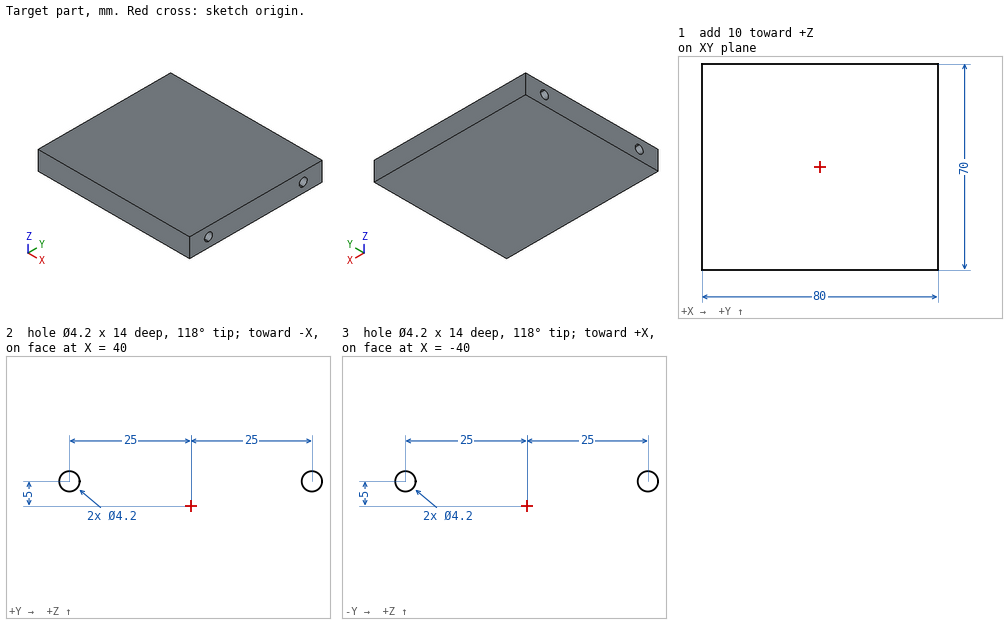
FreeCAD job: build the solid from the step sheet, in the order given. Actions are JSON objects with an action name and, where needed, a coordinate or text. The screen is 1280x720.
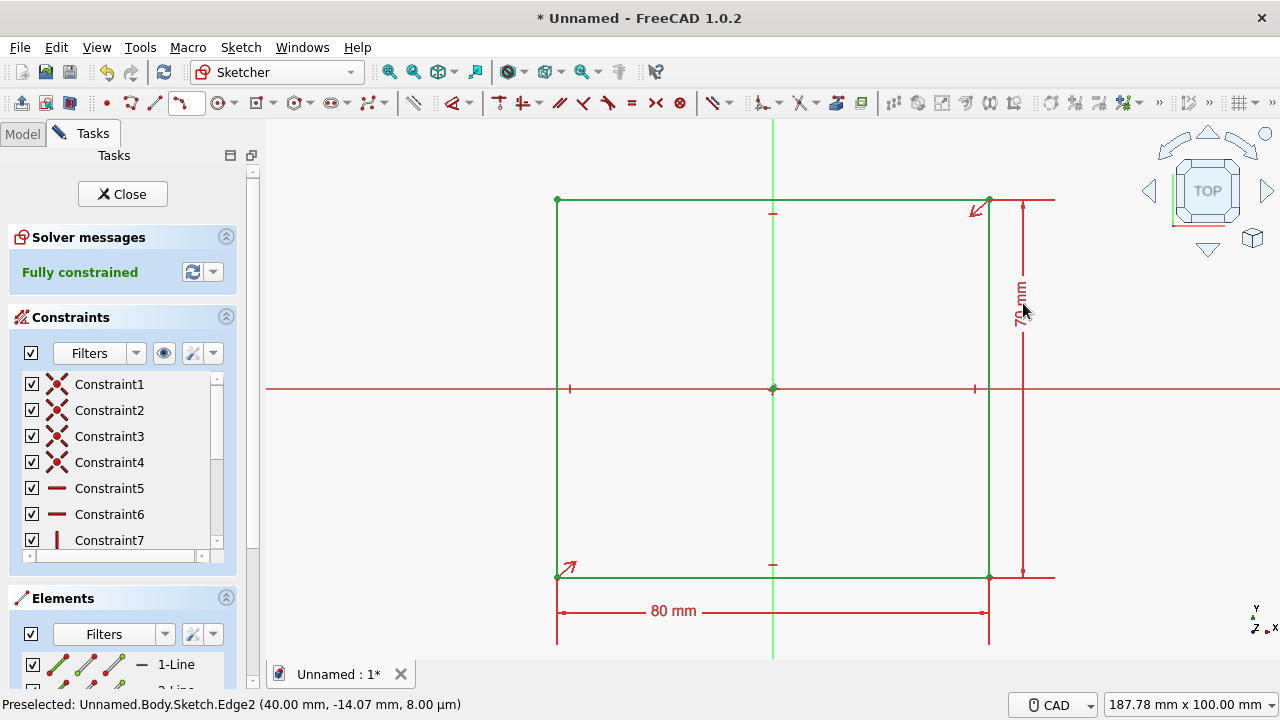
{"action": "left_click", "coordinate": [123, 194]}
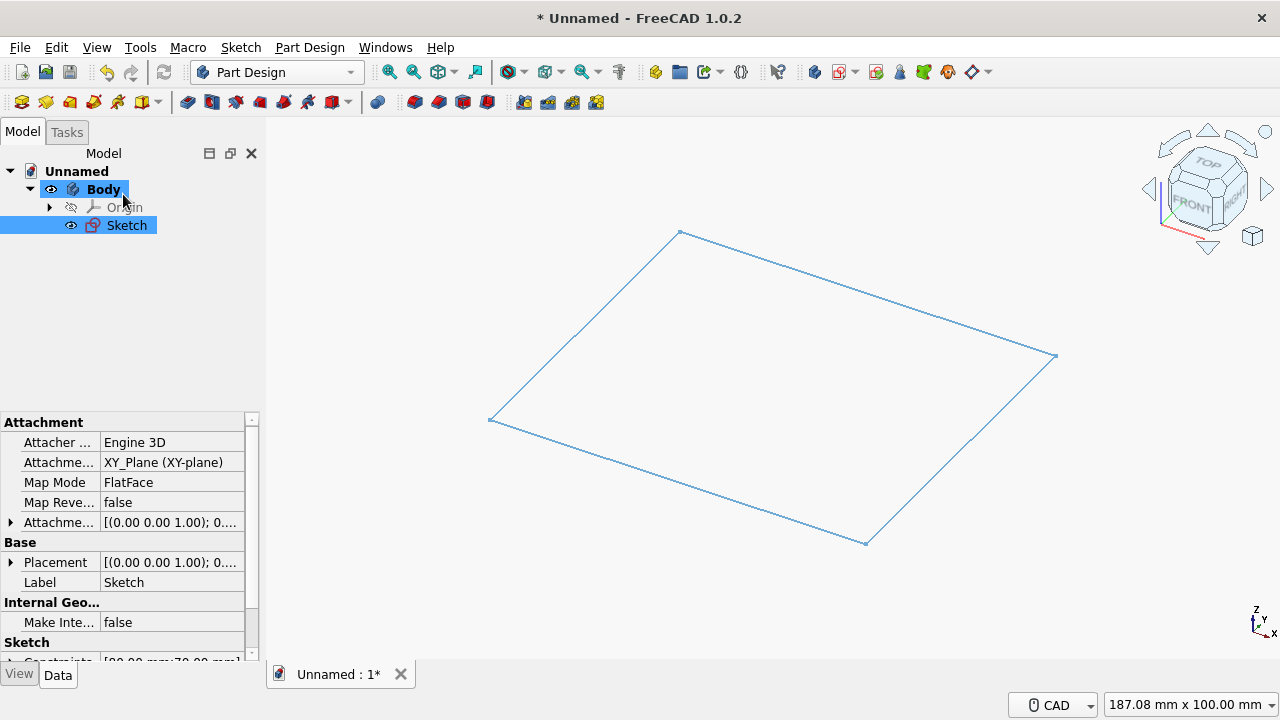
{"action": "left_click", "coordinate": [22, 102]}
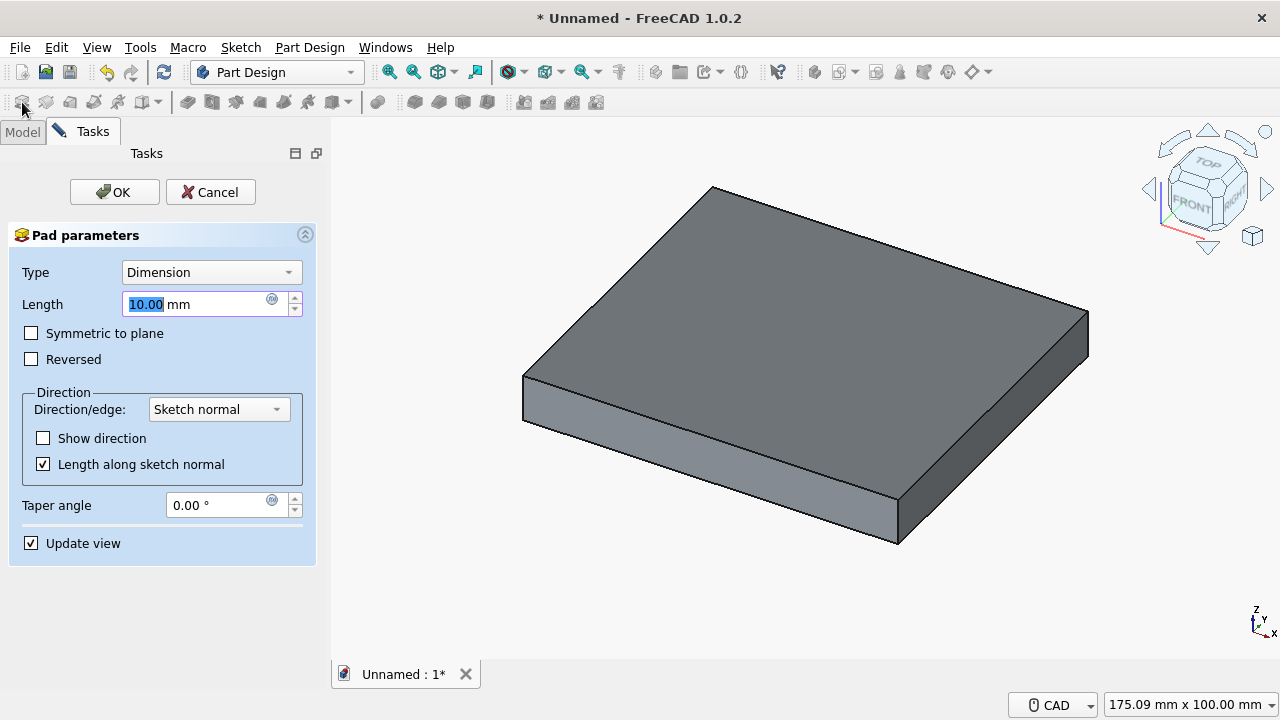
{"action": "type", "text": "10"}
{"action": "key", "text": "Tab"}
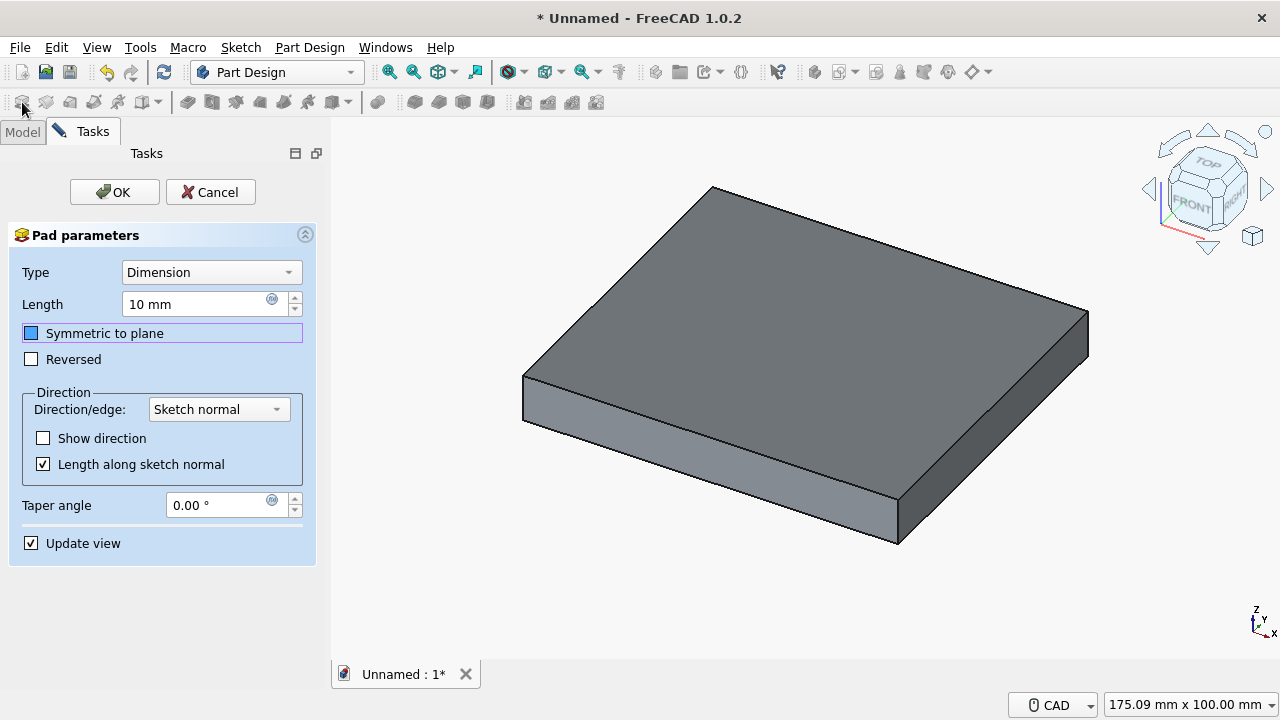
{"action": "left_click", "coordinate": [115, 192]}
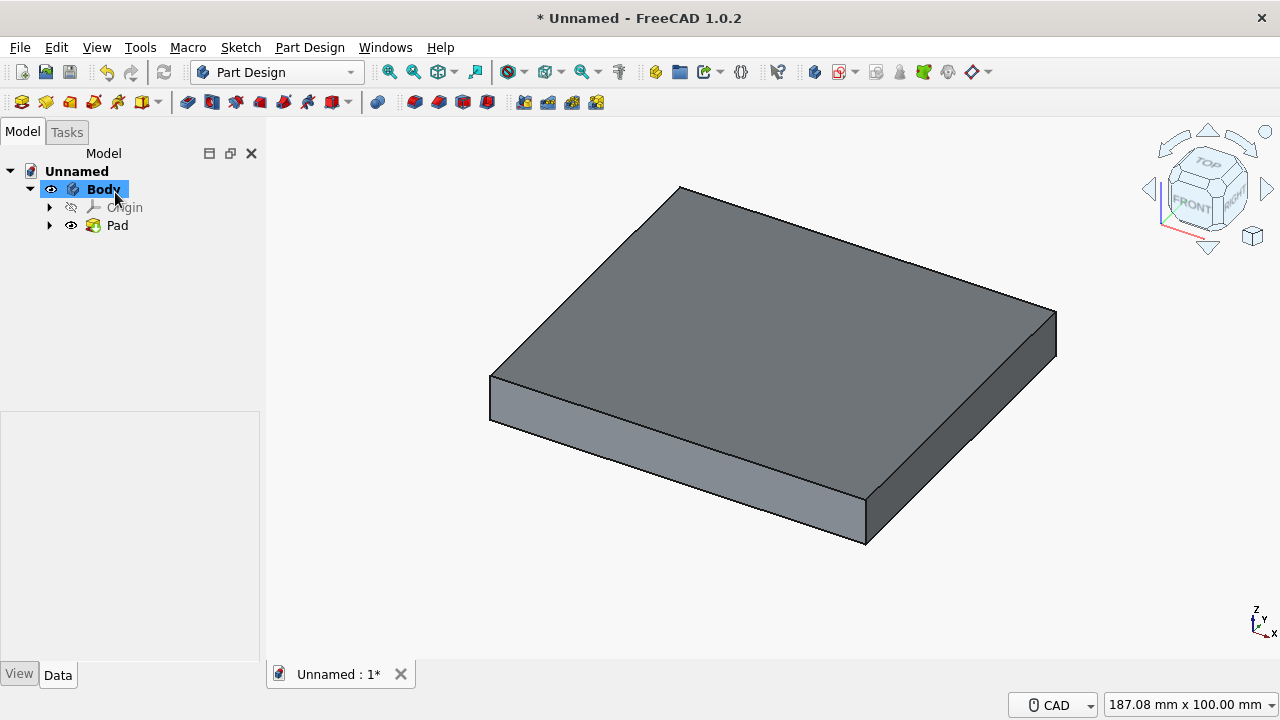
{"action": "left_click", "coordinate": [1042, 346]}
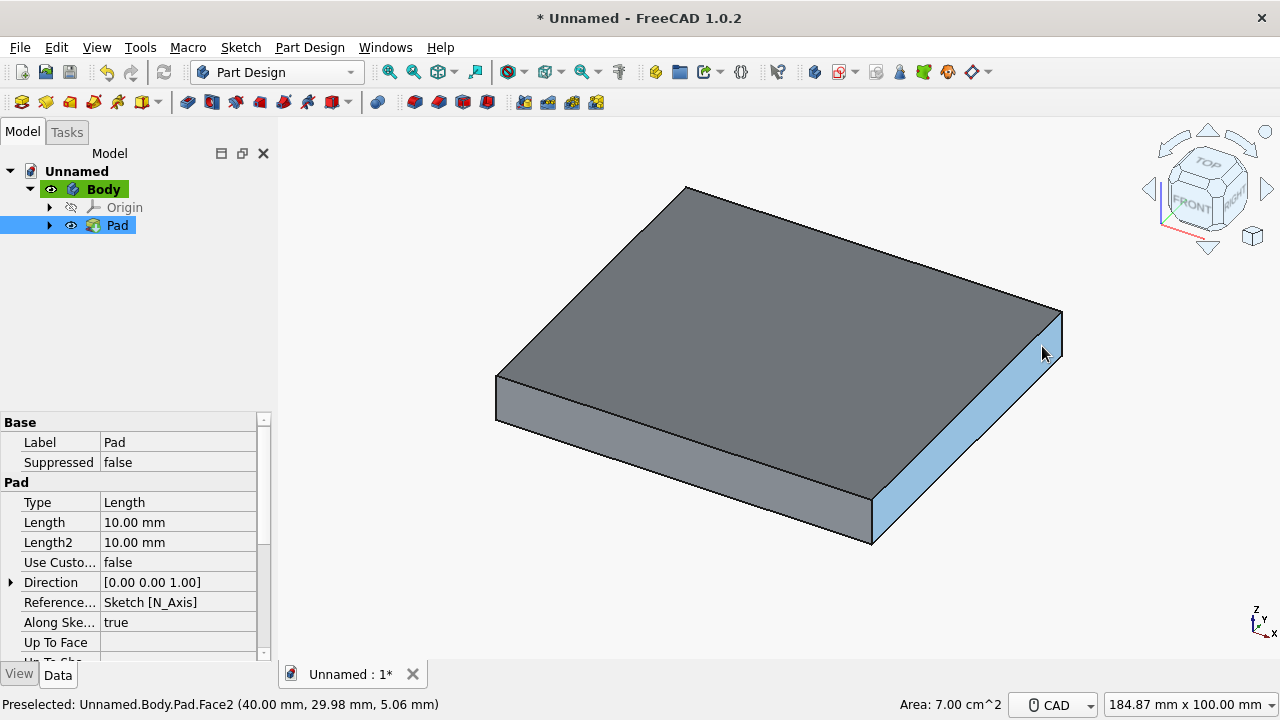
{"action": "left_click", "coordinate": [840, 72]}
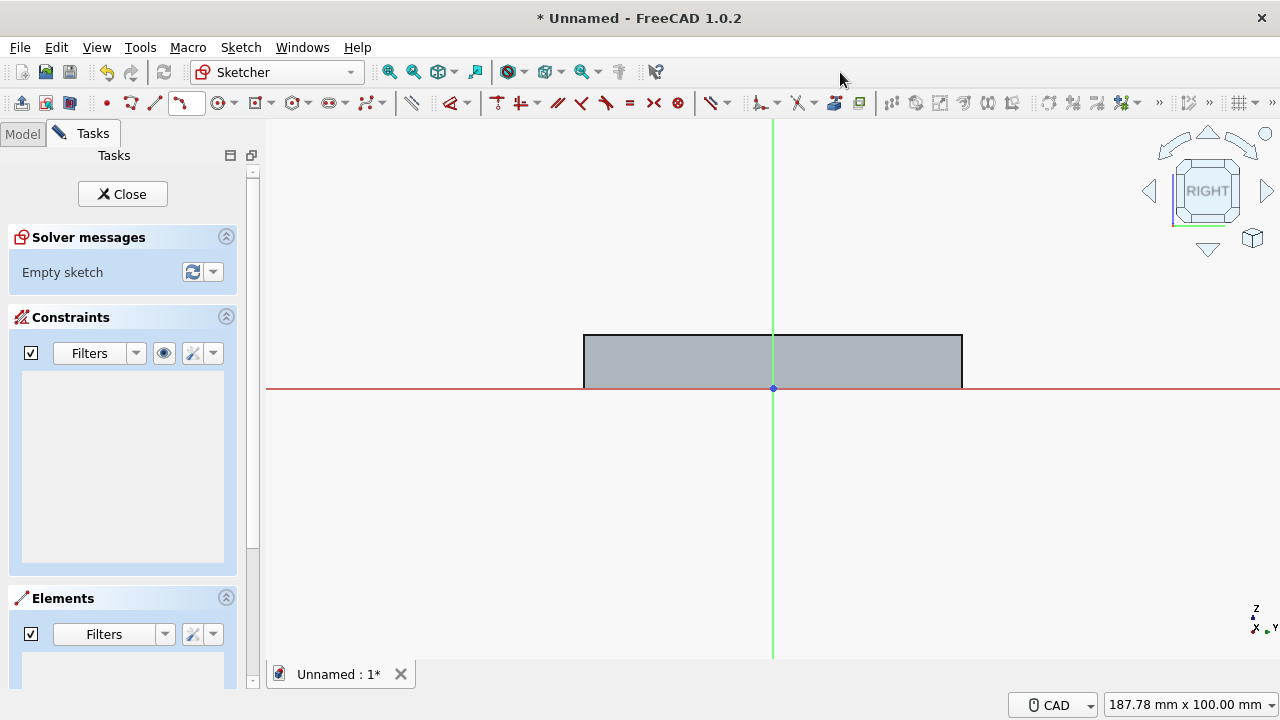
{"action": "scroll", "coordinate": [856, 347], "scroll_direction": "up", "scroll_amount": 3}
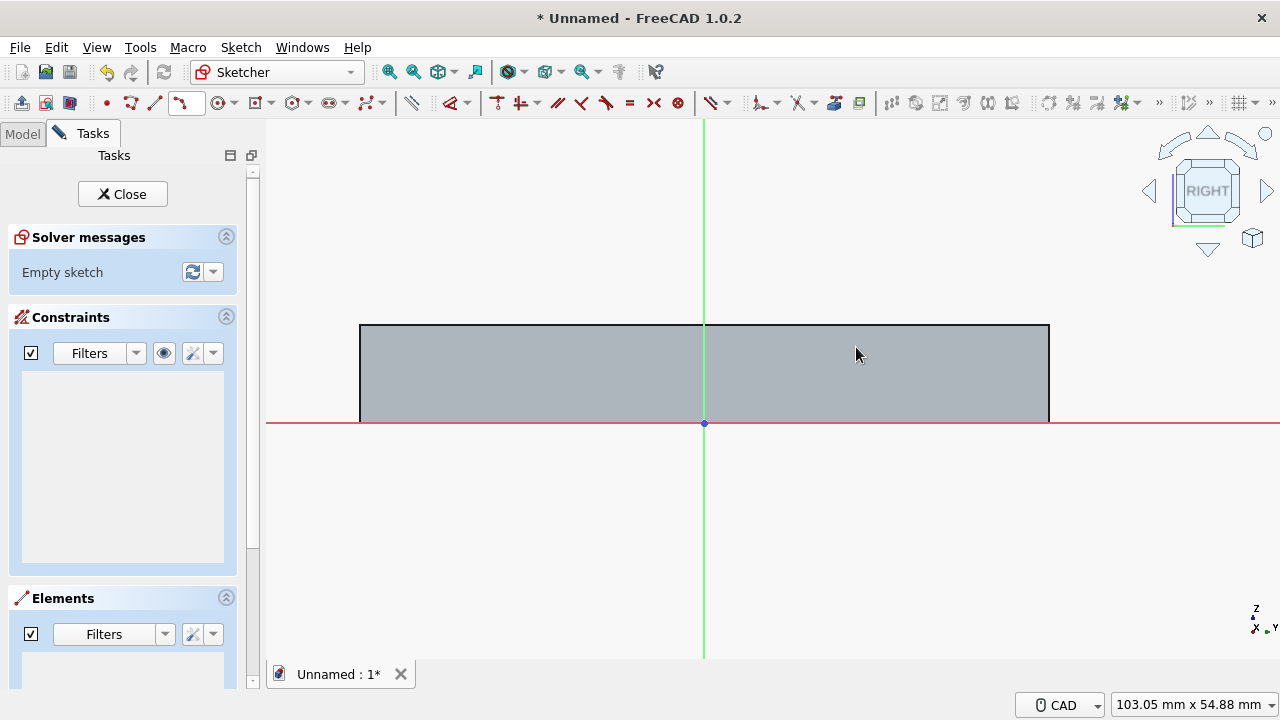
{"action": "left_click", "coordinate": [218, 104]}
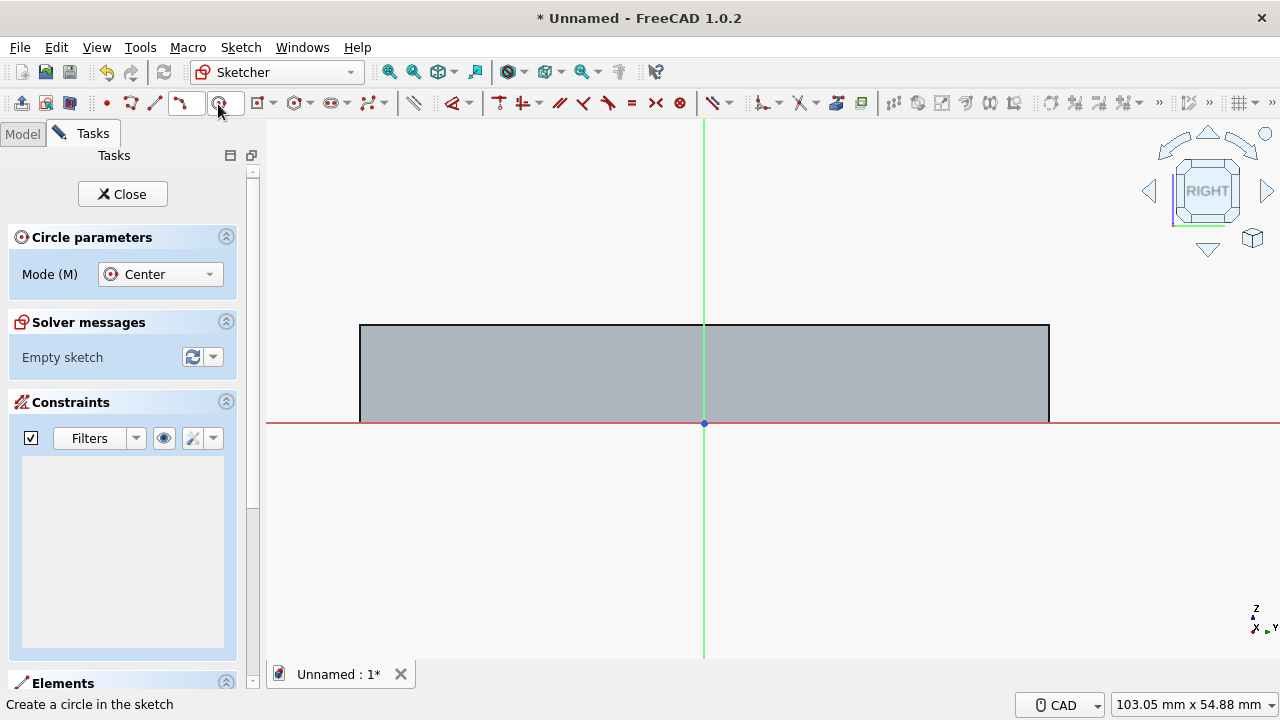
{"action": "left_click", "coordinate": [458, 374]}
{"action": "left_click", "coordinate": [473, 359]}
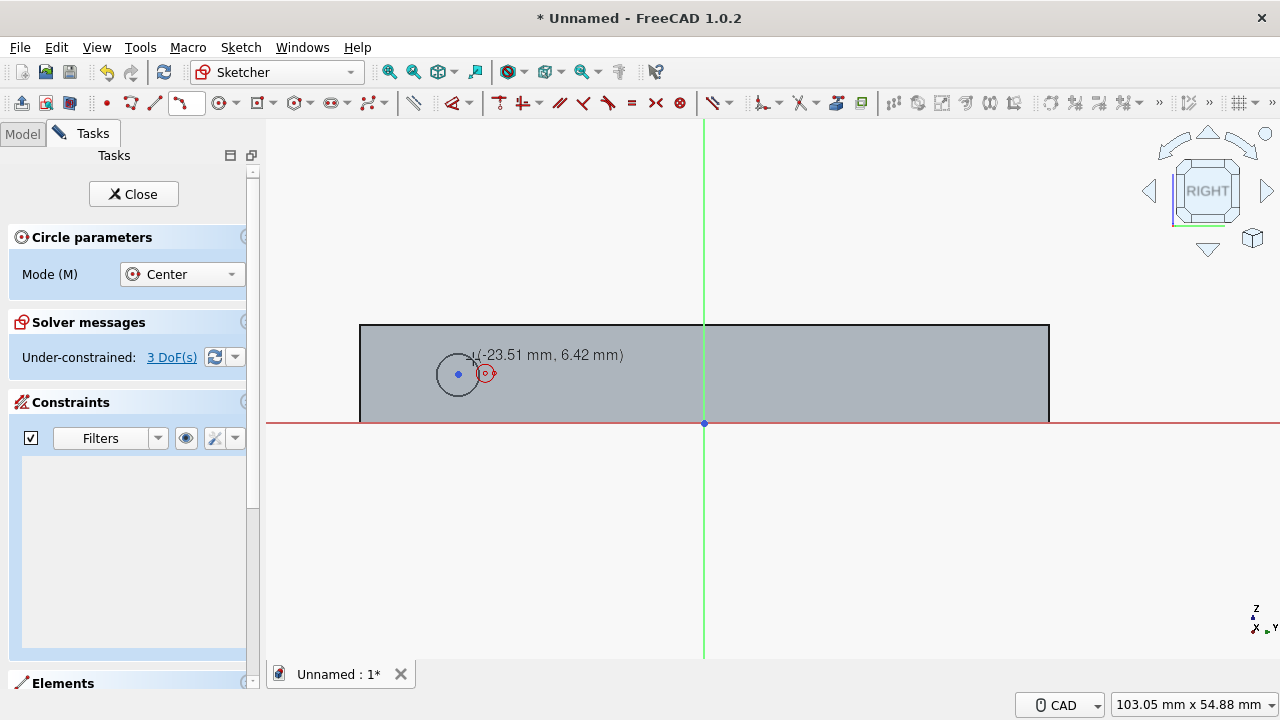
{"action": "left_click", "coordinate": [950, 374]}
{"action": "left_click", "coordinate": [965, 359]}
{"action": "key", "text": "Escape"}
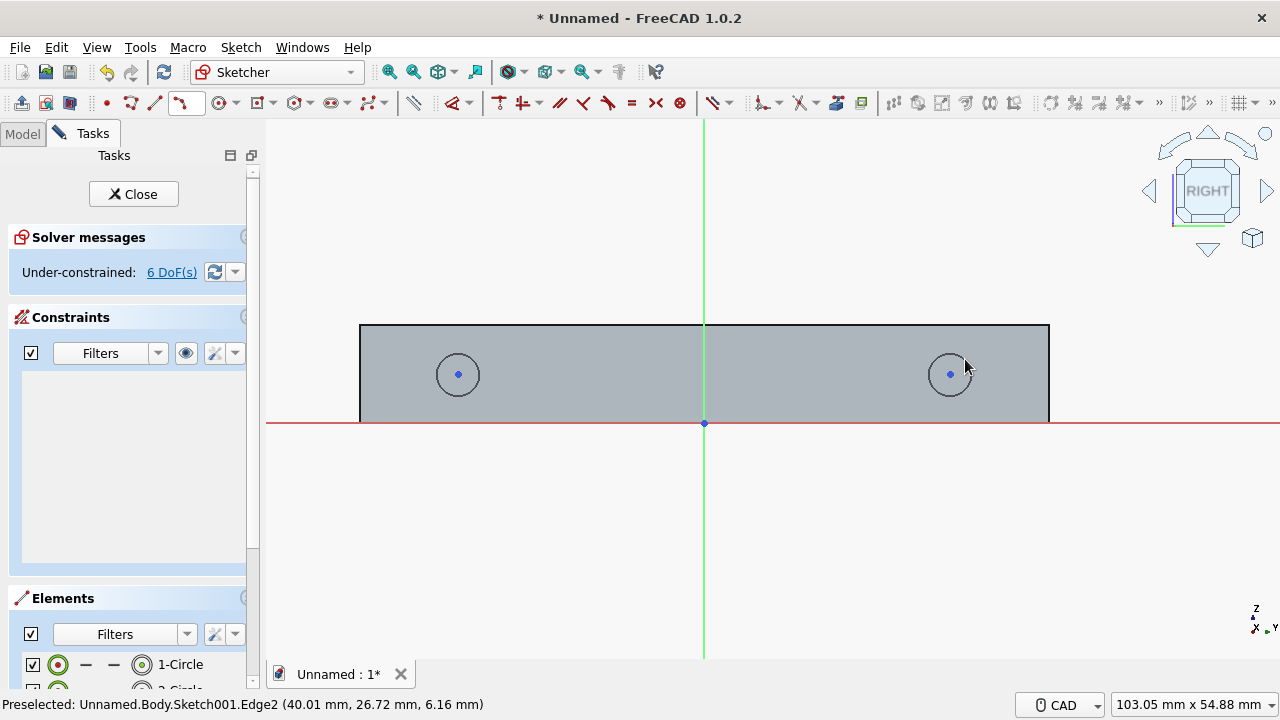
{"action": "left_click", "coordinate": [473, 360]}